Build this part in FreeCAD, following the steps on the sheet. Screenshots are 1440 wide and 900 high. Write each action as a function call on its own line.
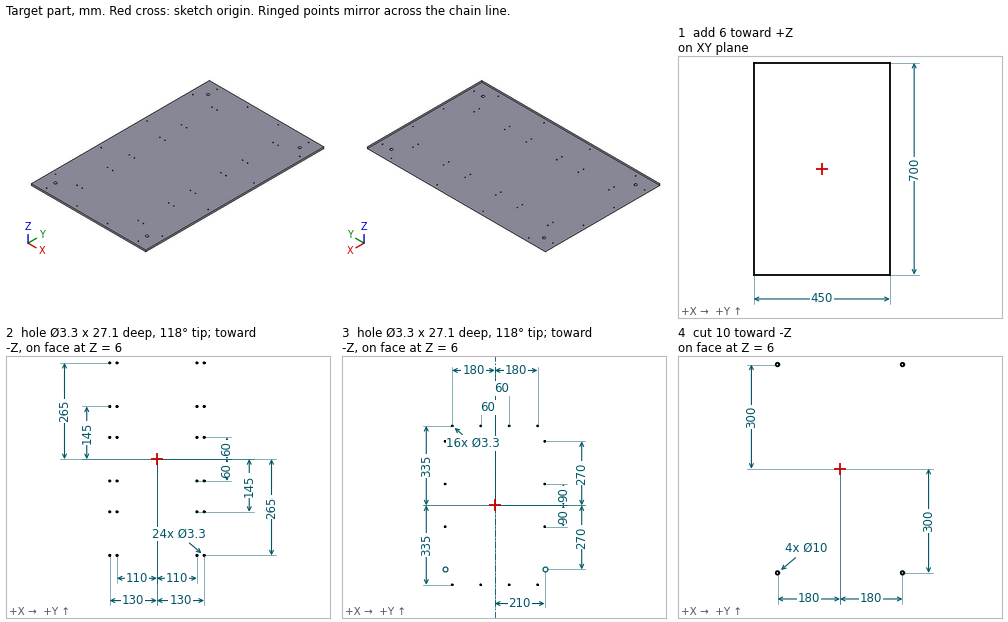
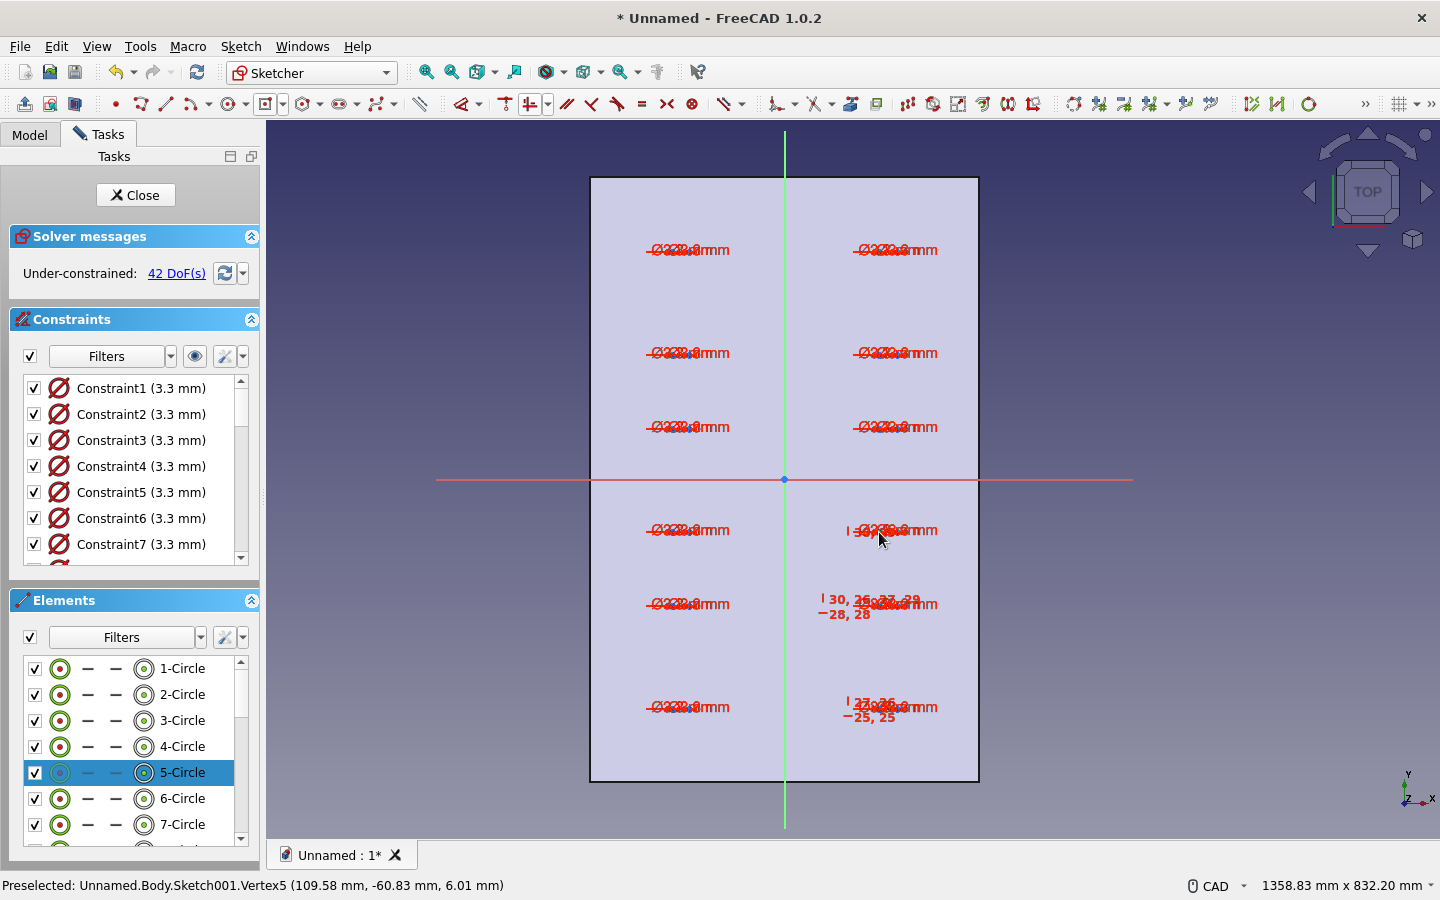
click(897, 532)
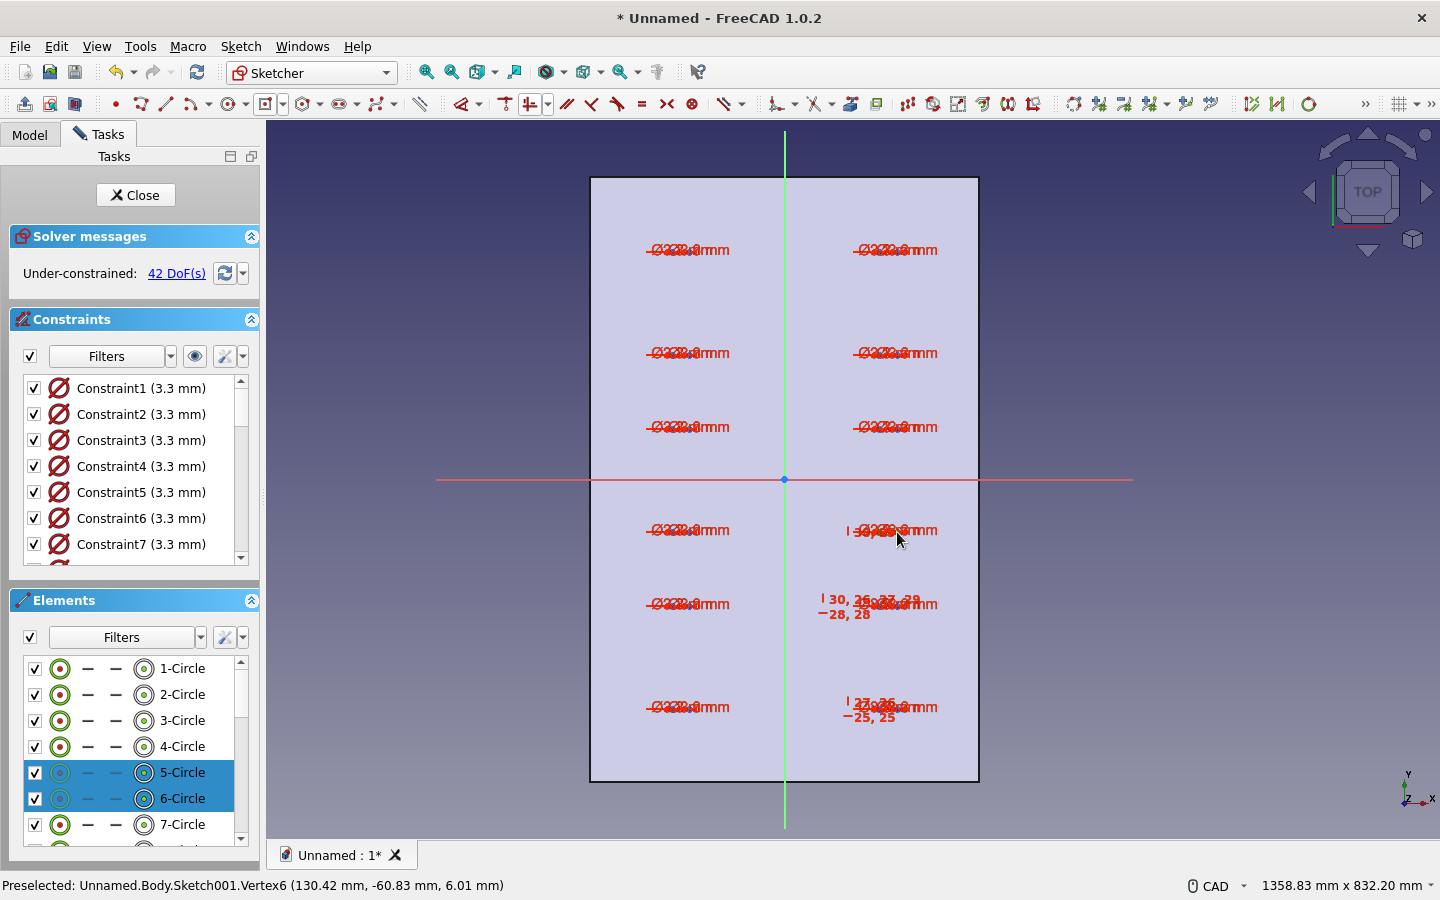
click(548, 104)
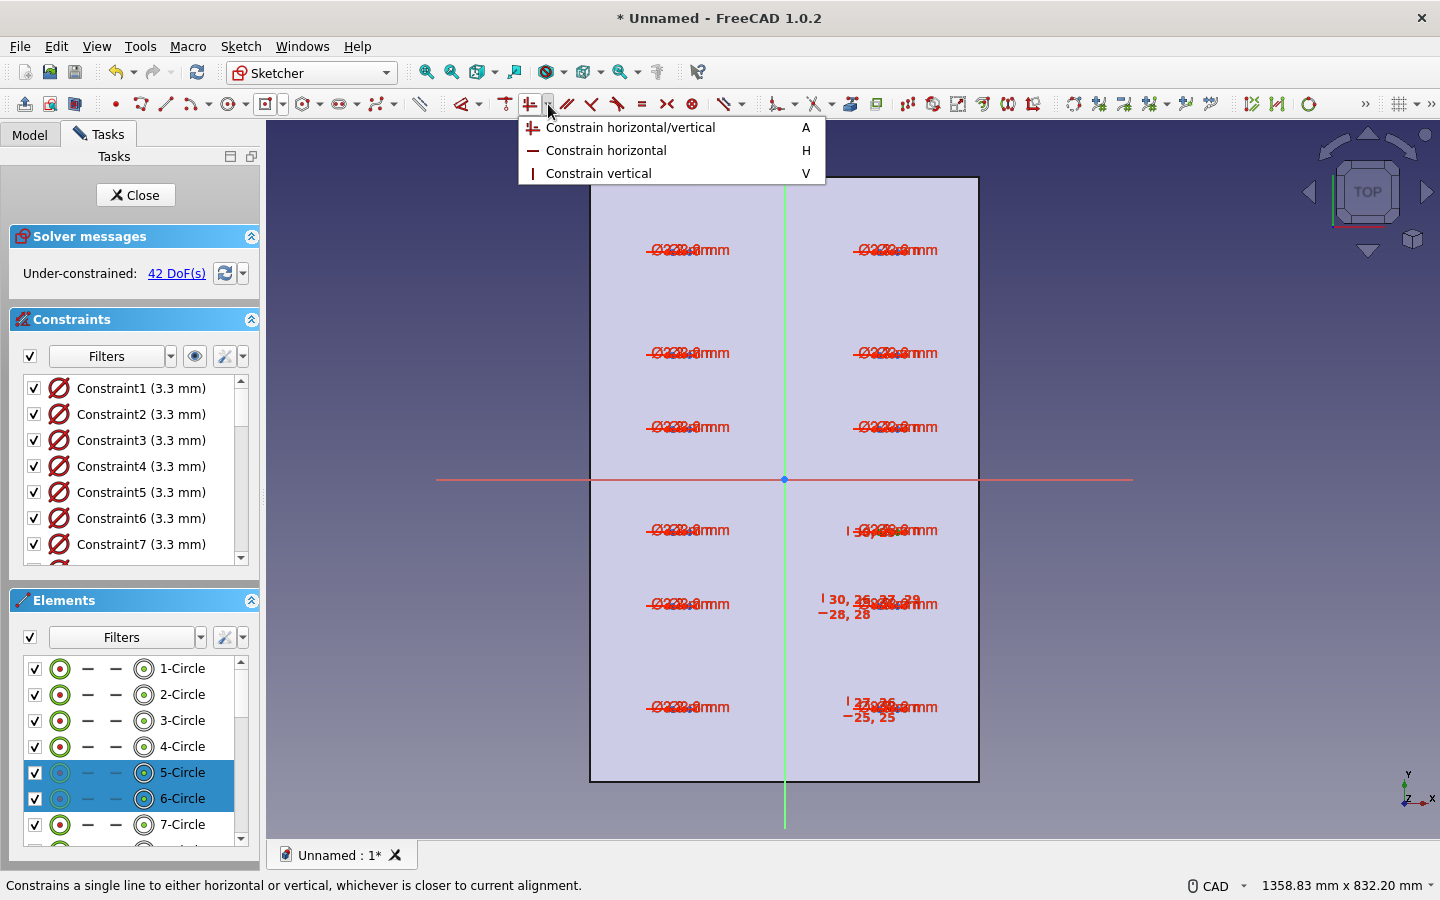
click(672, 150)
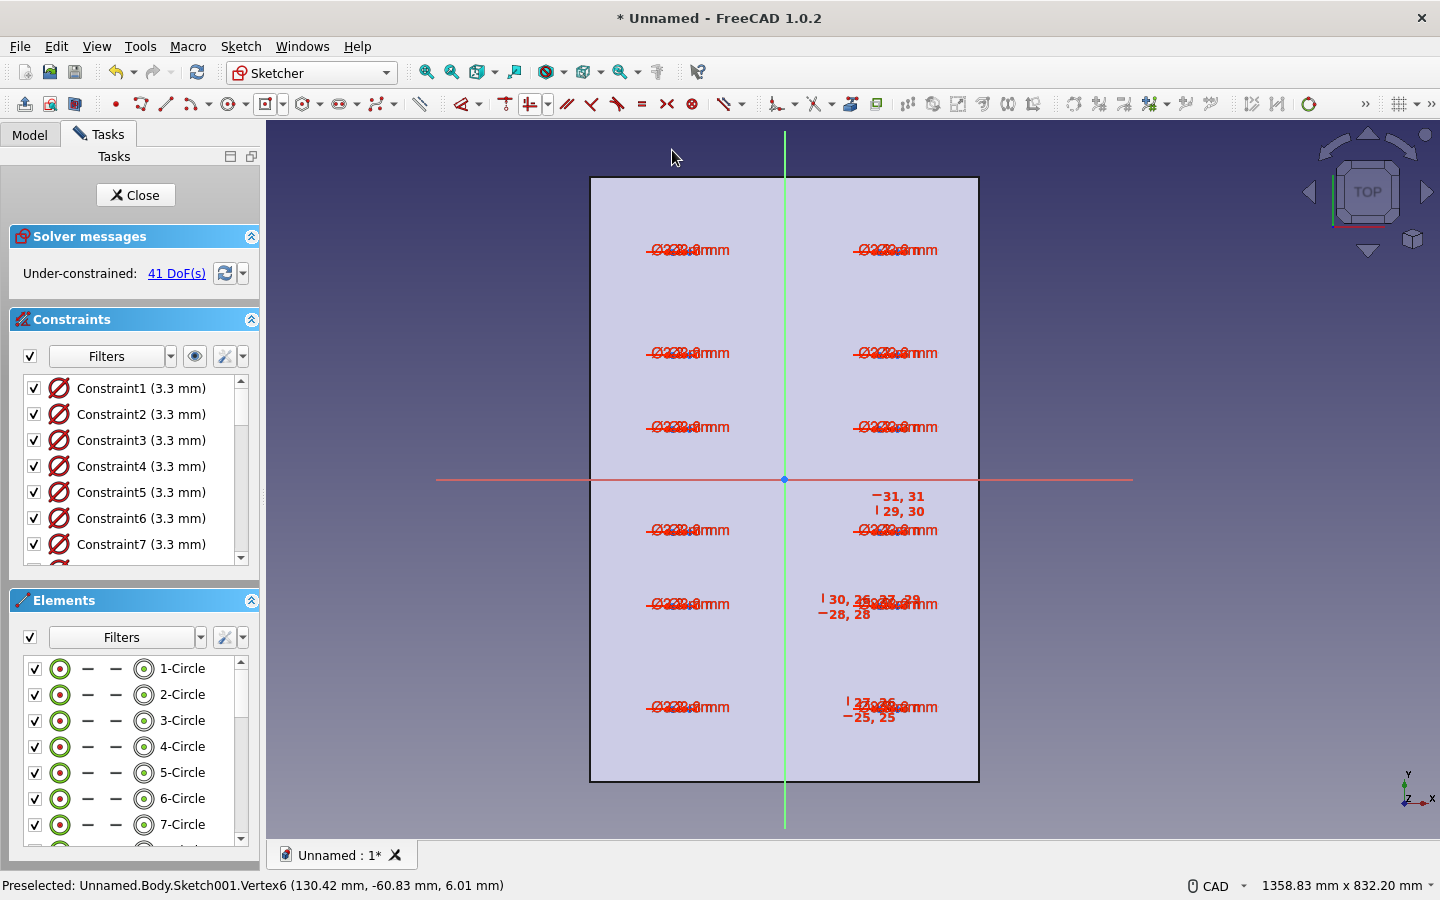
click(897, 532)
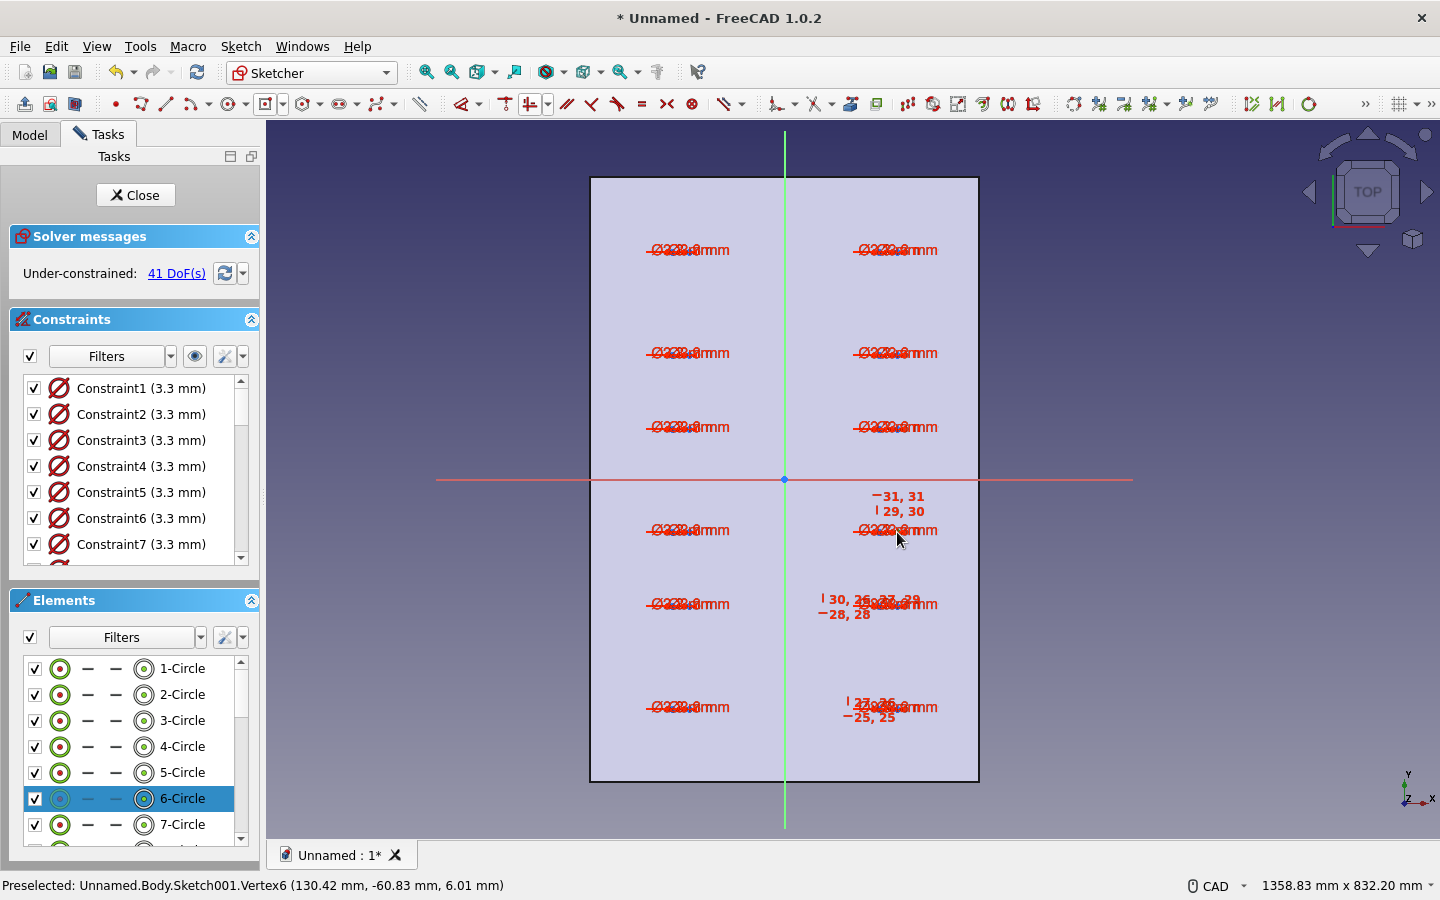
click(897, 429)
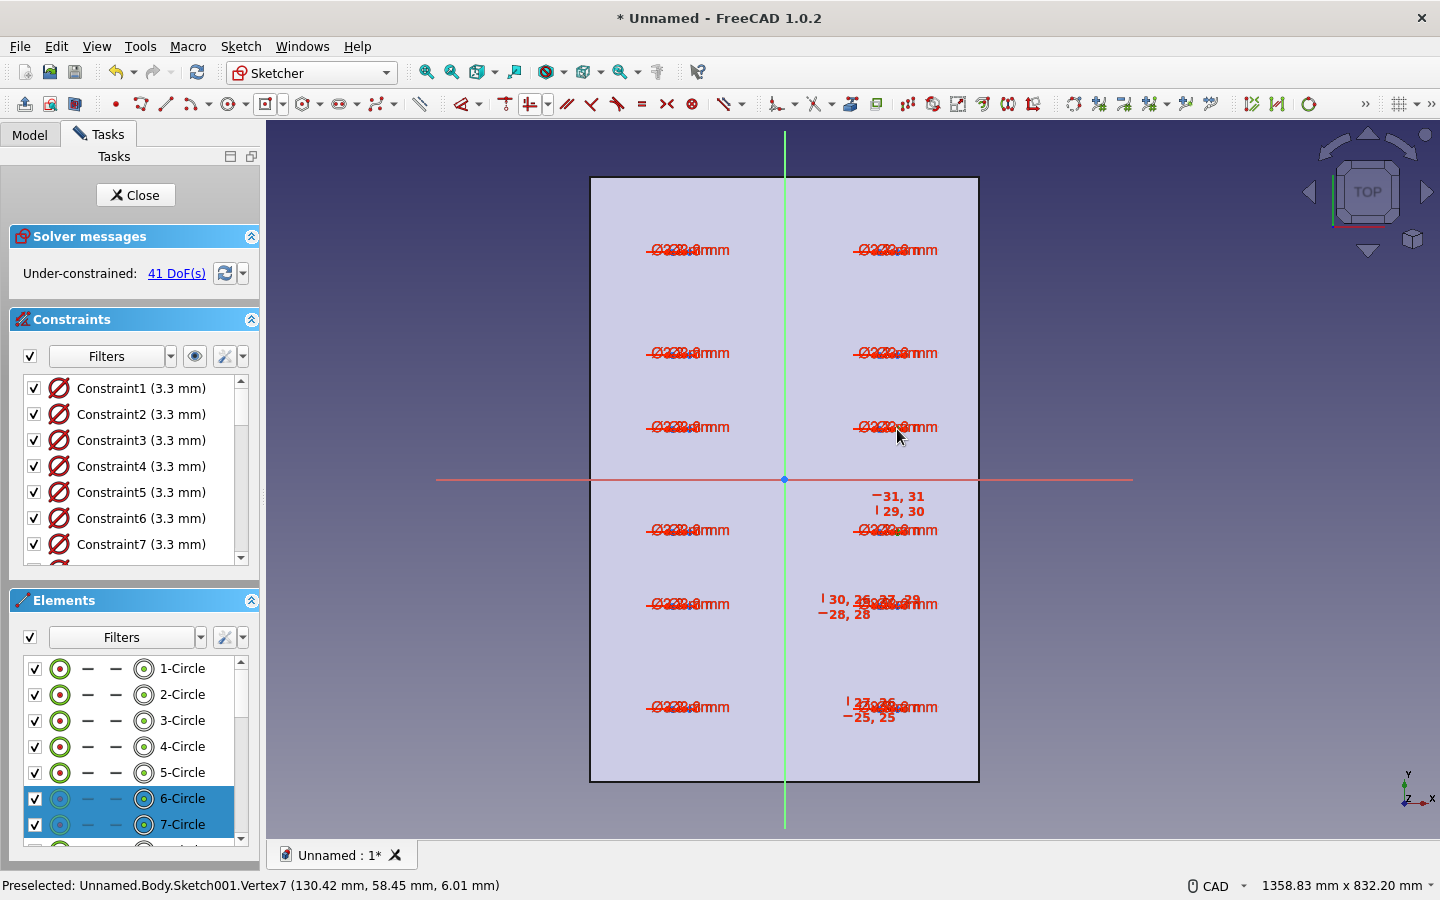
key(v)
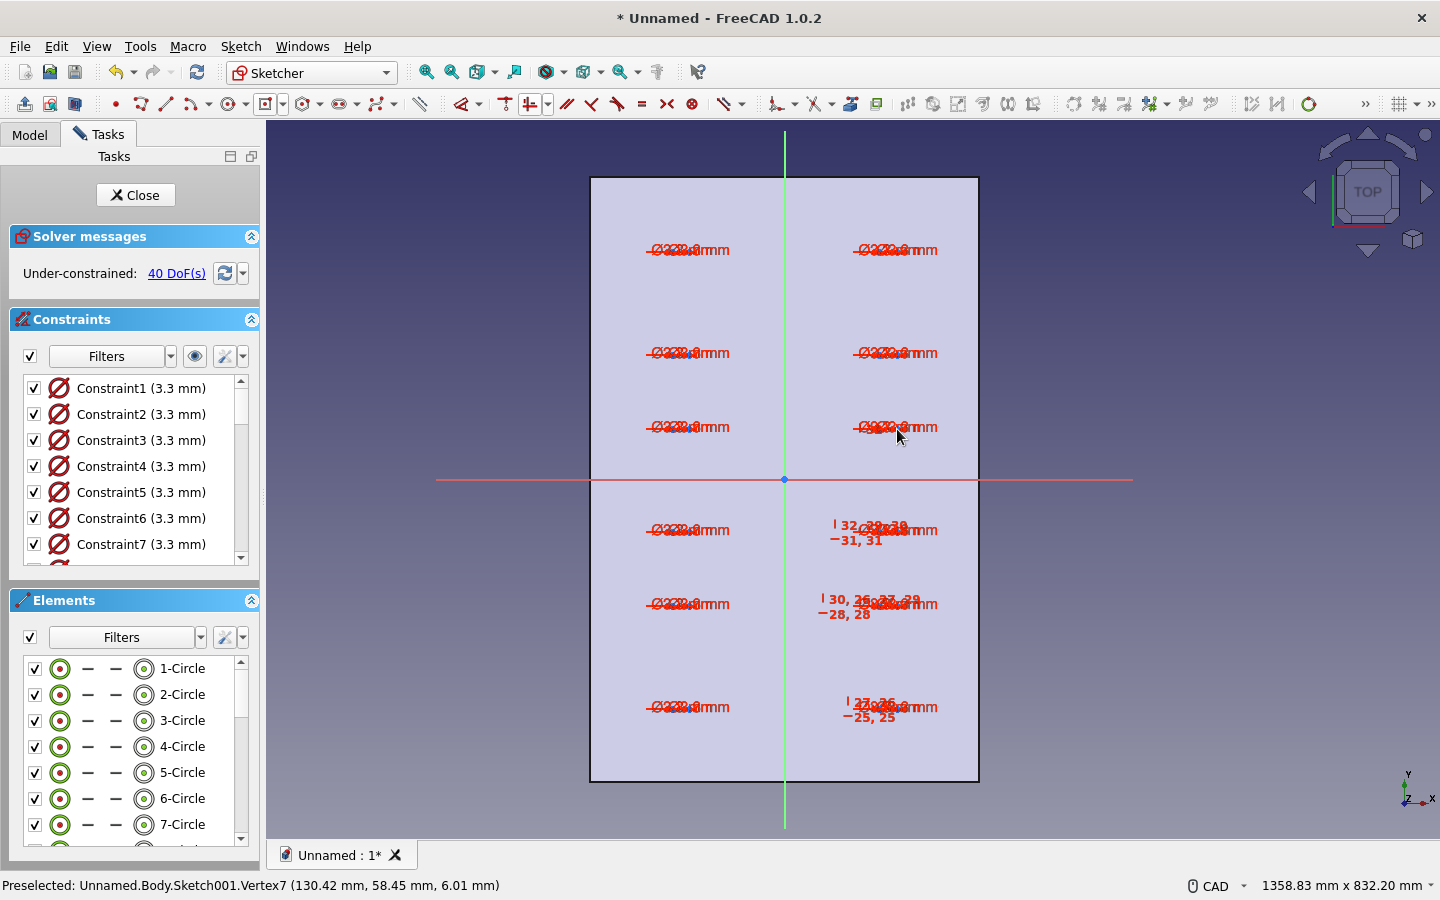
click(879, 532)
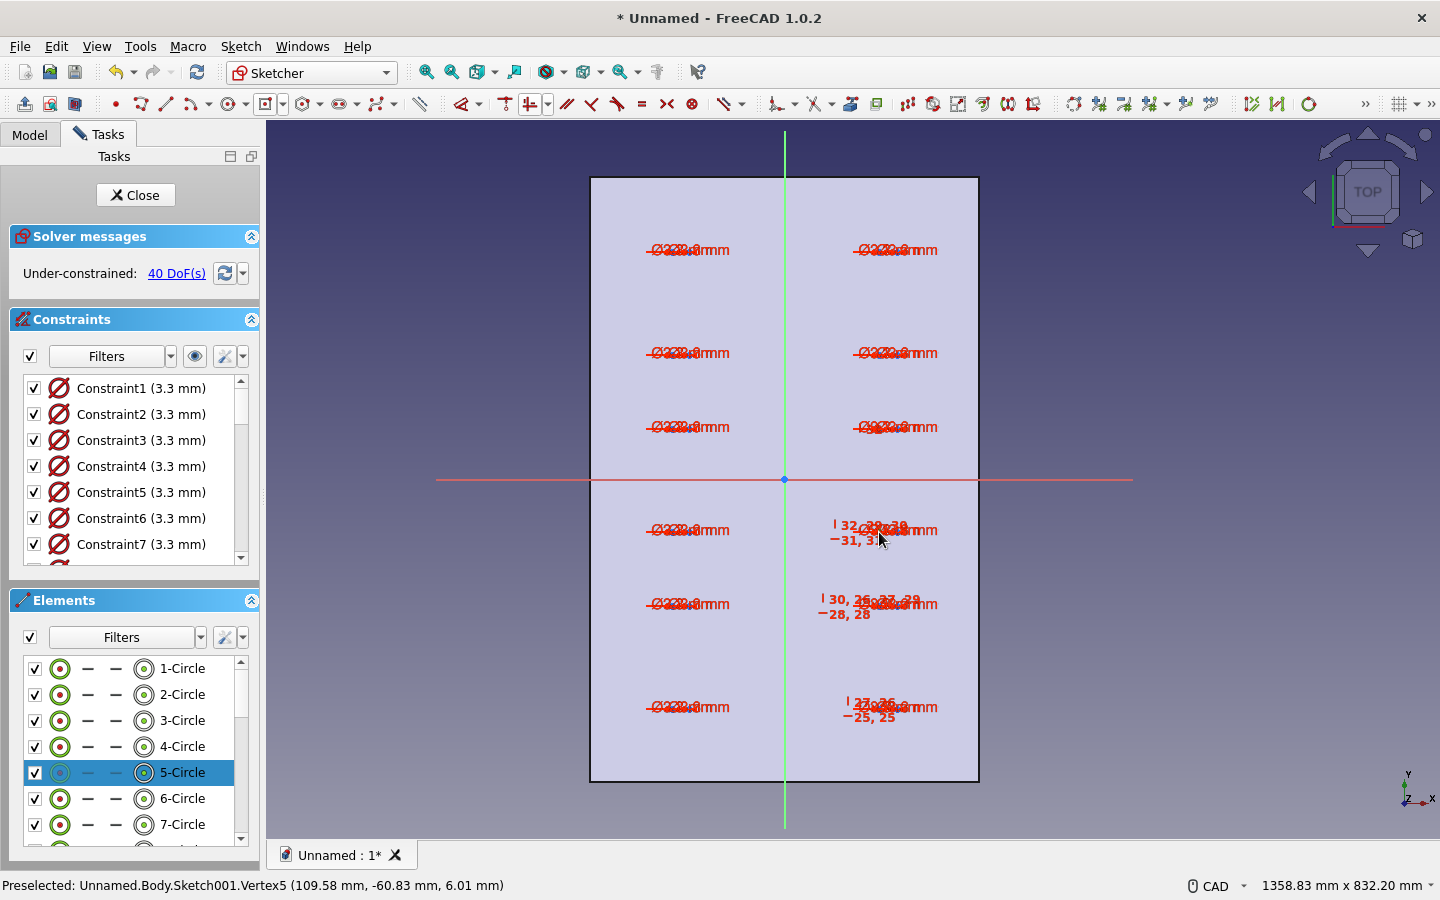
scroll(879, 429, up, 4)